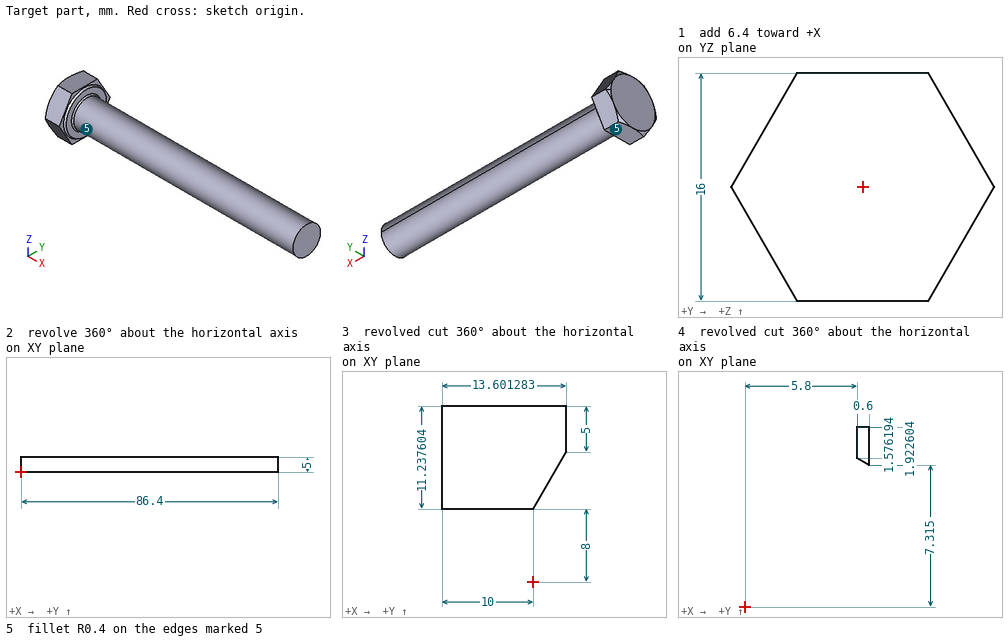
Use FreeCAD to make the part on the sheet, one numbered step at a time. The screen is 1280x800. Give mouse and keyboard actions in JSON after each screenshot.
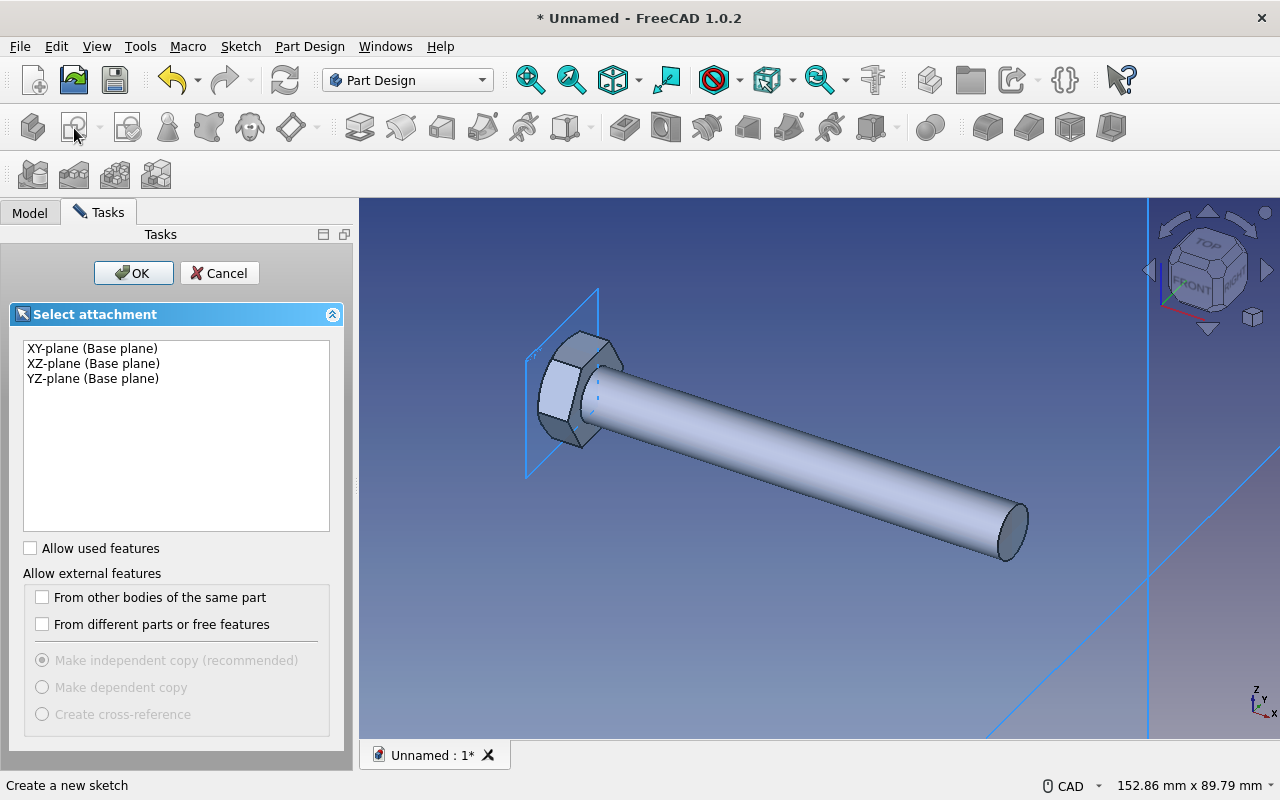
{"action": "left_click", "coordinate": [84, 348]}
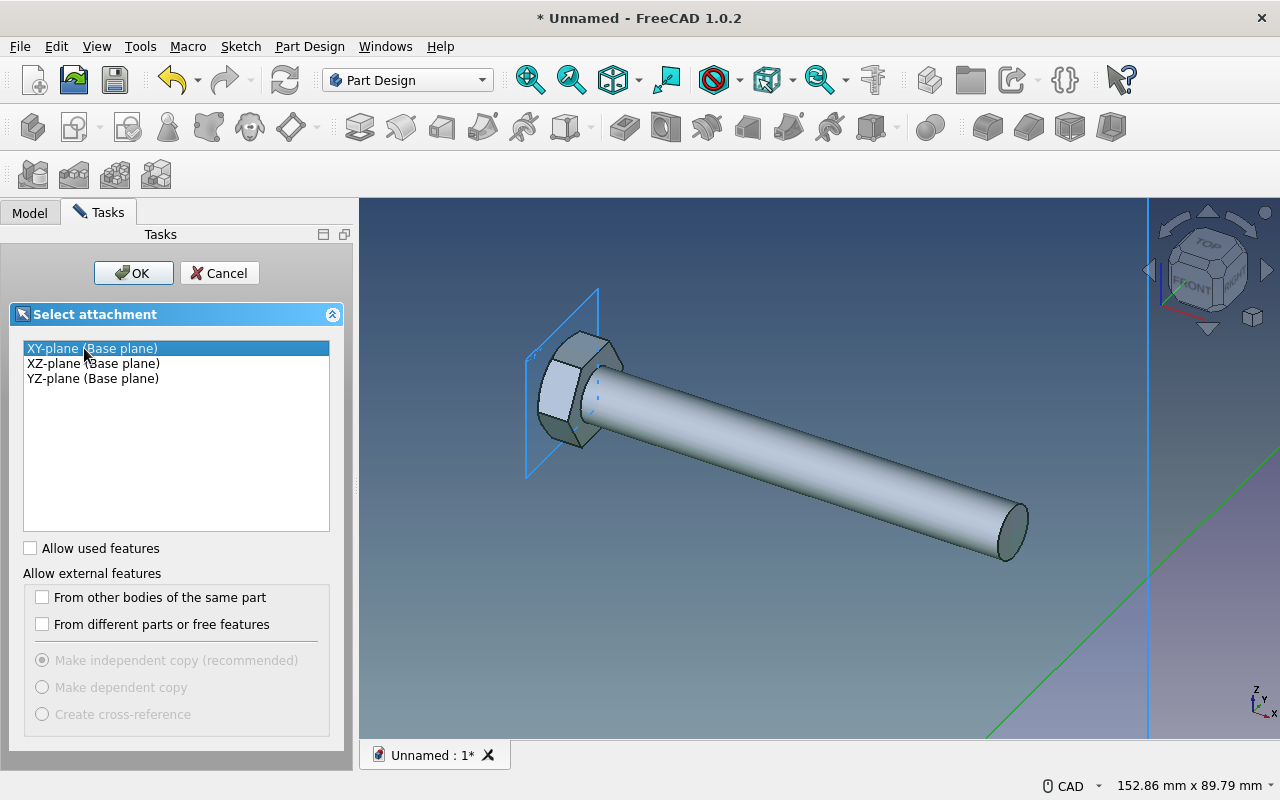
{"action": "left_click", "coordinate": [134, 273]}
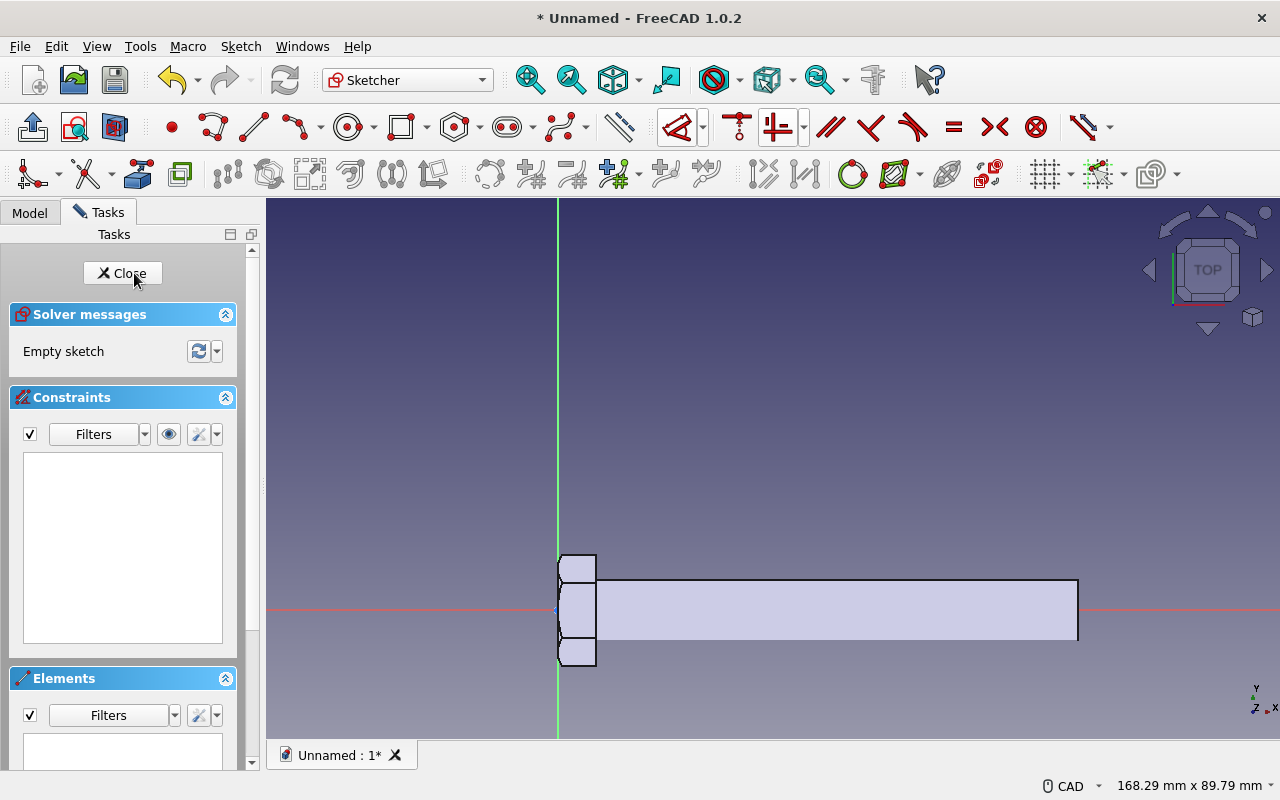
{"action": "left_click", "coordinate": [115, 128]}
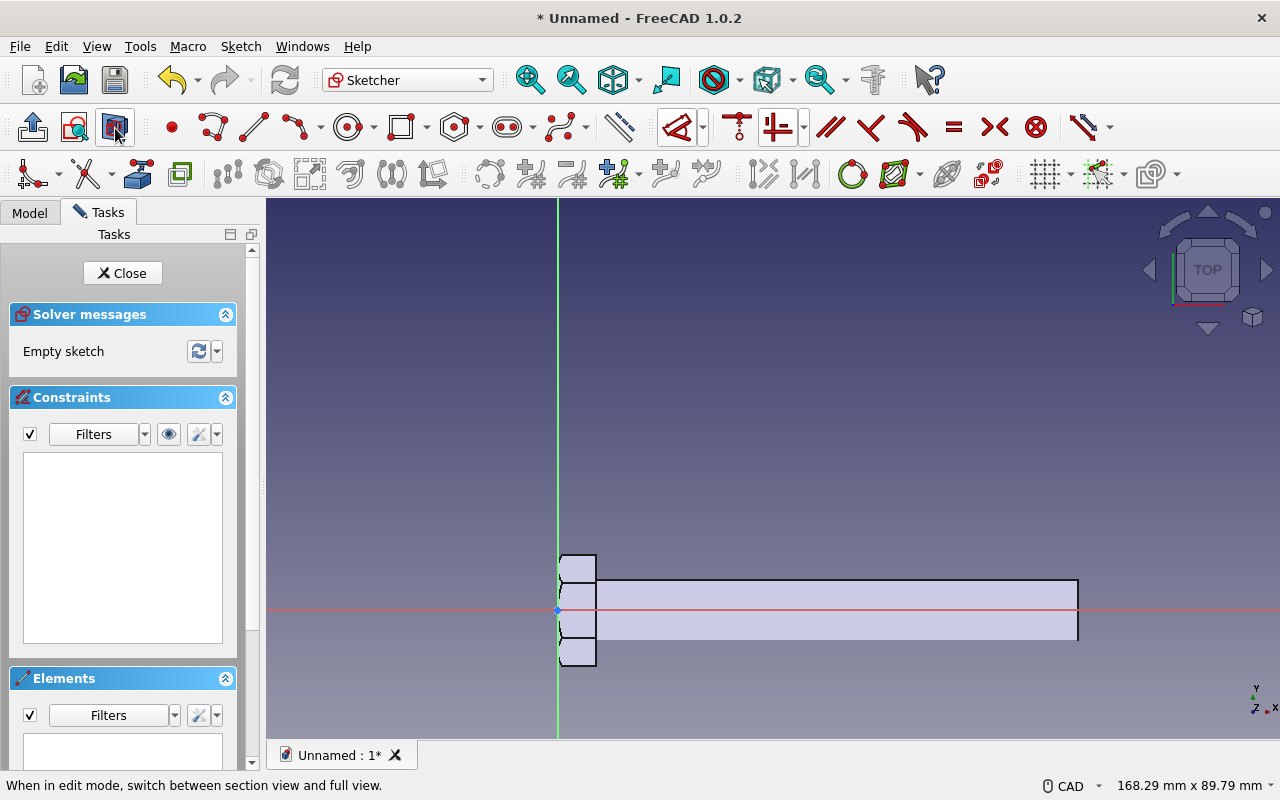
{"action": "scroll", "coordinate": [589, 565], "scroll_direction": "up", "scroll_amount": 15}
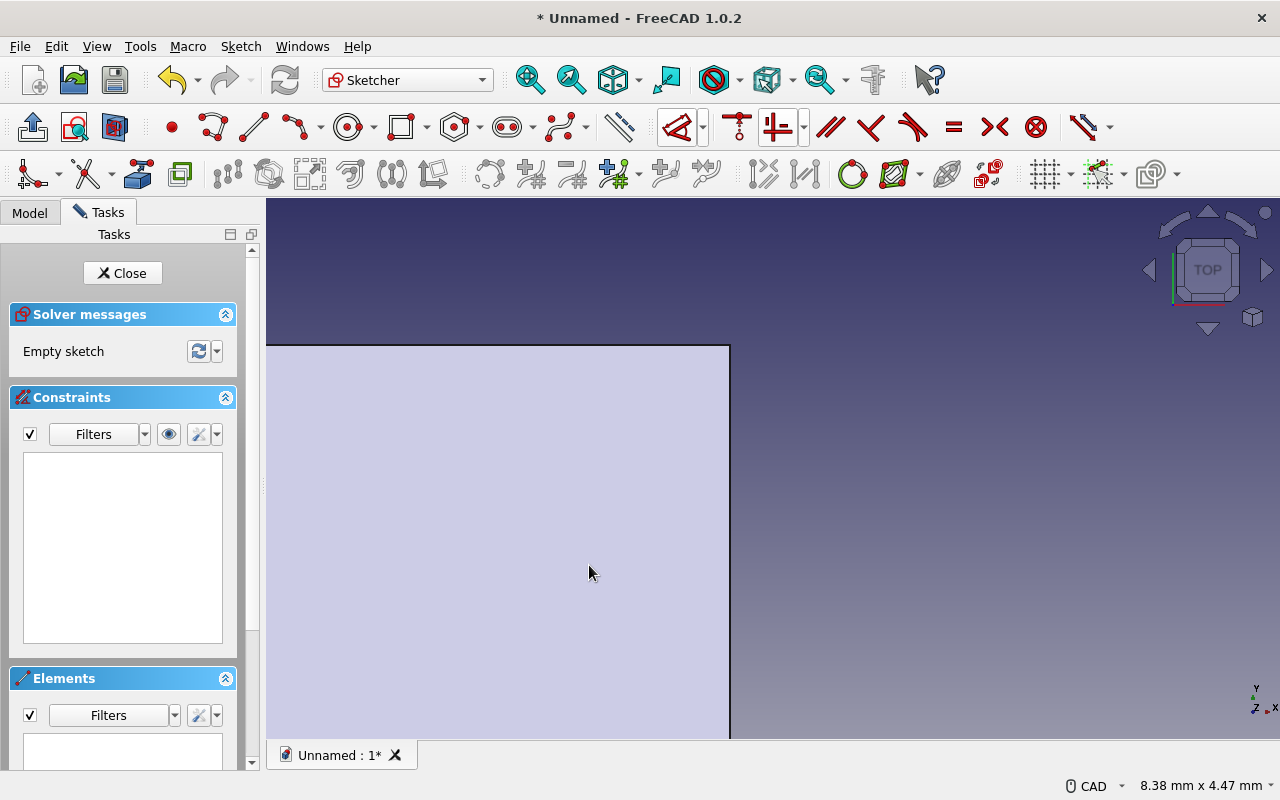
{"action": "scroll", "coordinate": [671, 446], "scroll_direction": "up", "scroll_amount": 2}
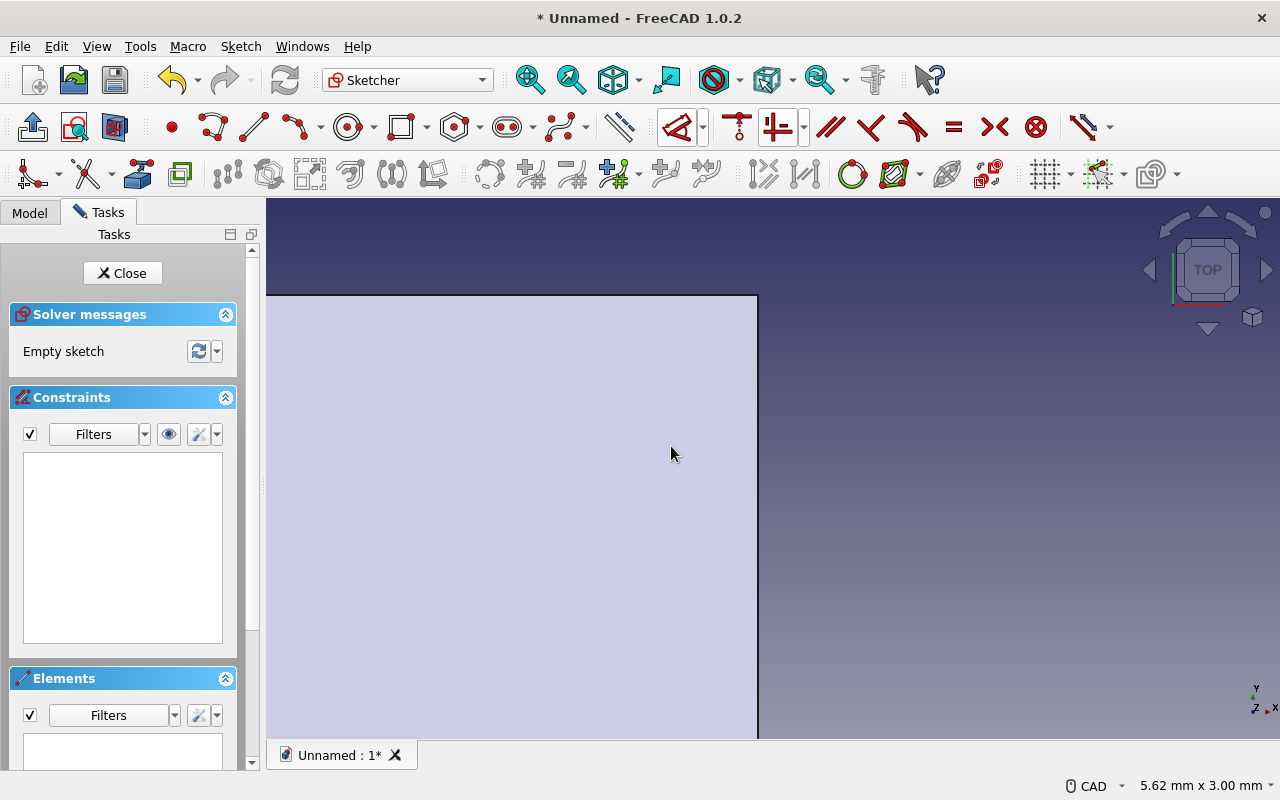
{"action": "key", "text": "g m"}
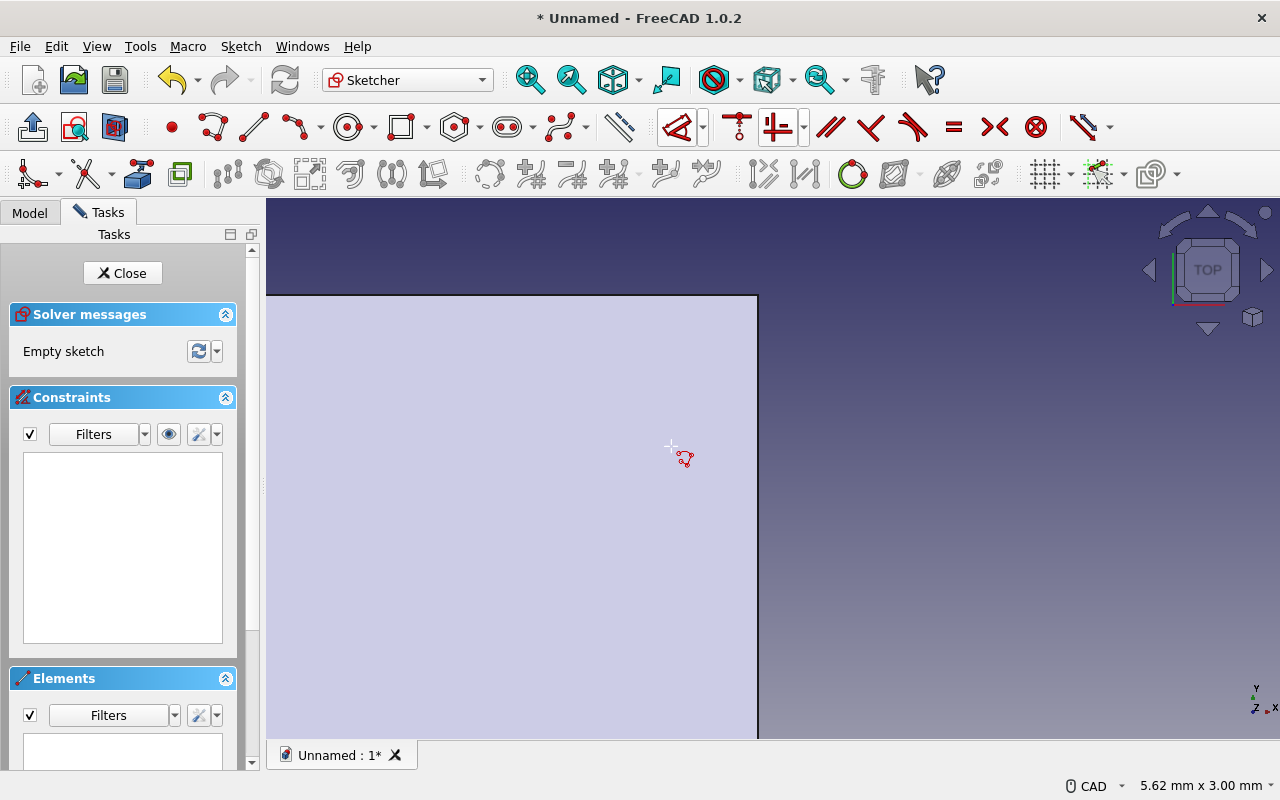
{"action": "left_click", "coordinate": [650, 579]}
{"action": "left_click", "coordinate": [758, 642]}
{"action": "left_click", "coordinate": [758, 295]}
{"action": "left_click", "coordinate": [650, 295]}
{"action": "left_click", "coordinate": [650, 580]}
{"action": "key", "text": "Escape"}
{"action": "key", "text": "Escape"}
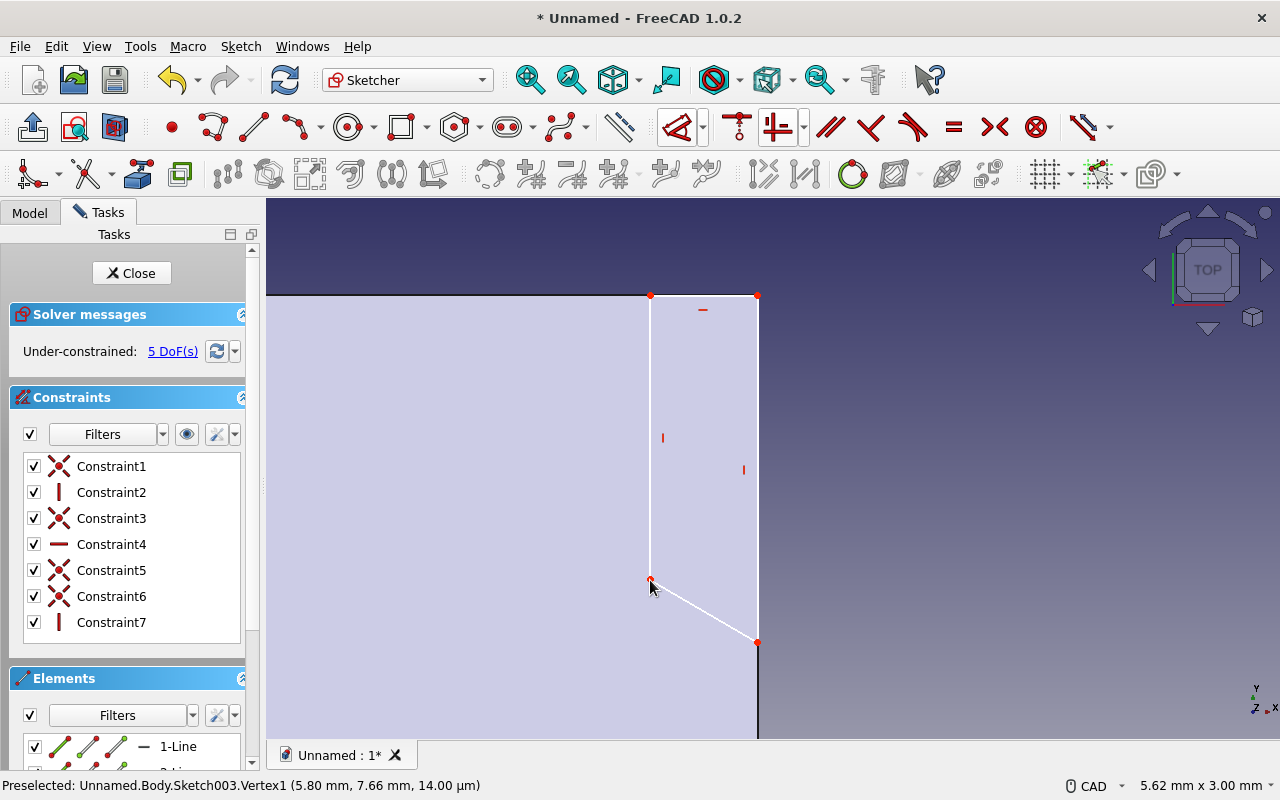
{"action": "left_click", "coordinate": [726, 296]}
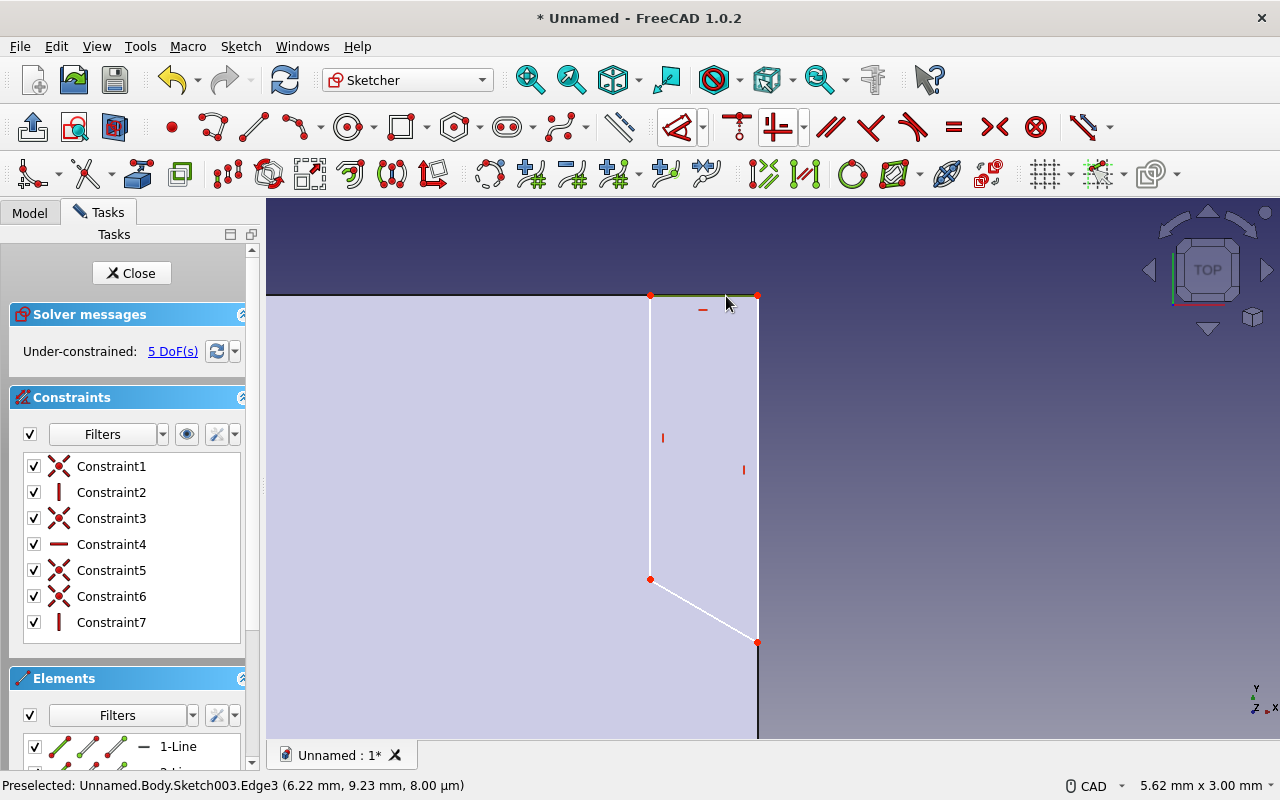
{"action": "left_click", "coordinate": [702, 128]}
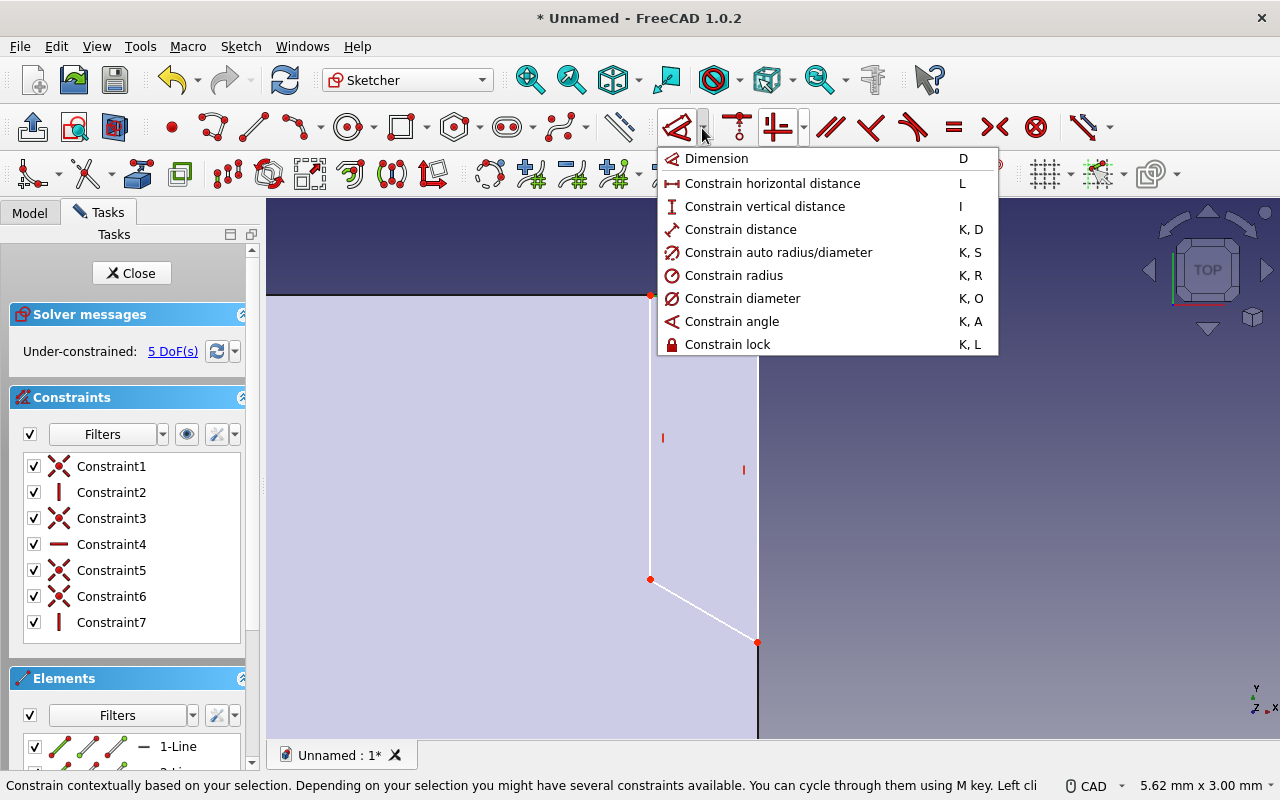
{"action": "left_click", "coordinate": [828, 184]}